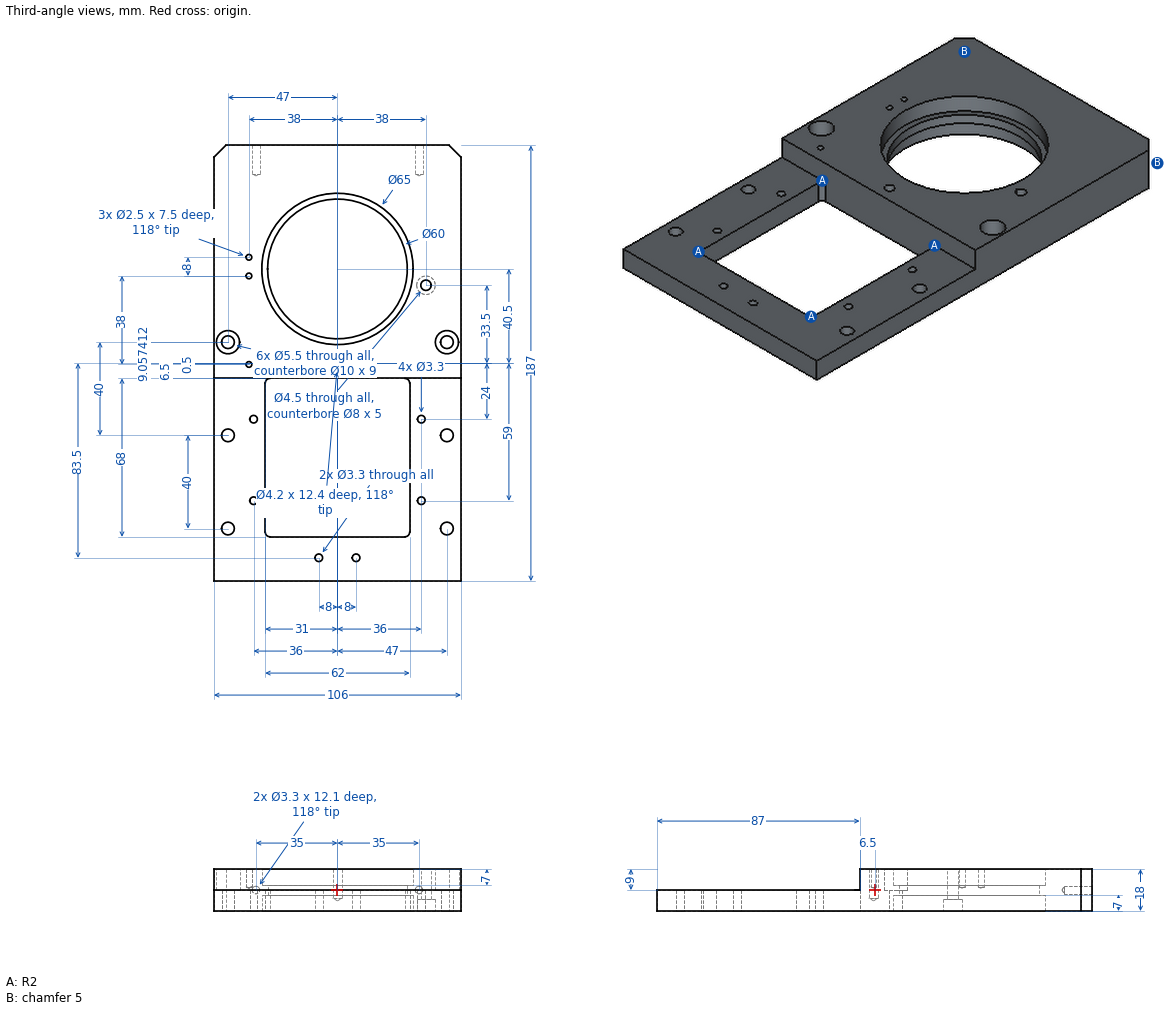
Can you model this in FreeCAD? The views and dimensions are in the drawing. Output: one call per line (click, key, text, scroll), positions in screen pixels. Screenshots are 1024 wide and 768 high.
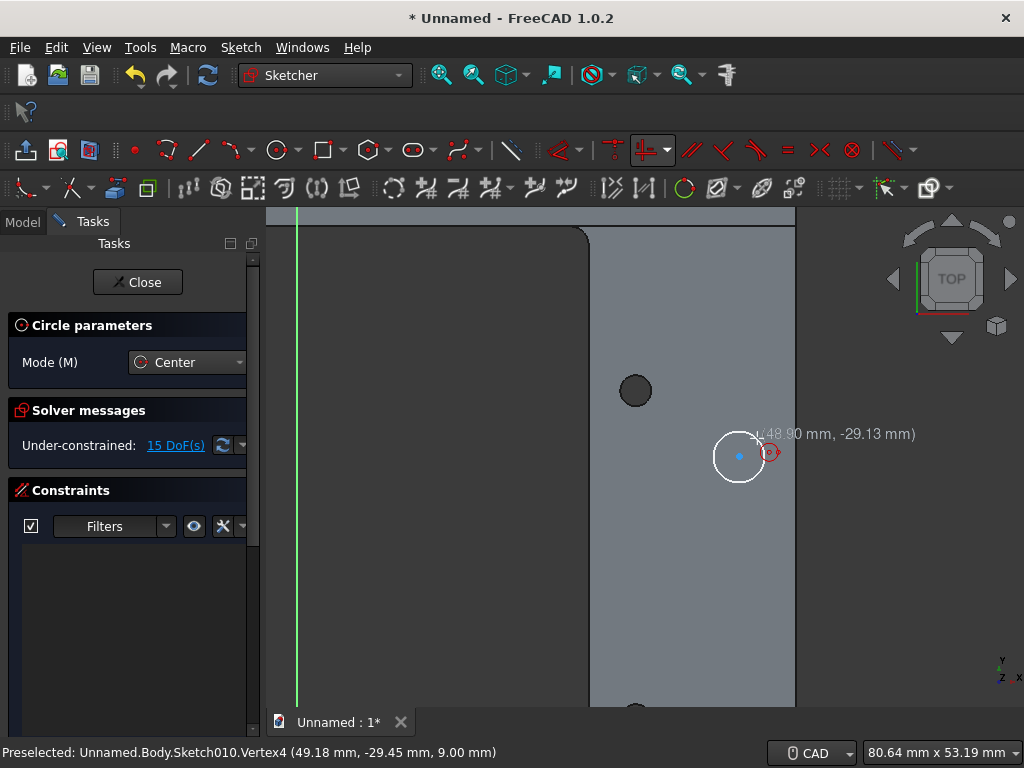
scroll(739, 458, down, 5)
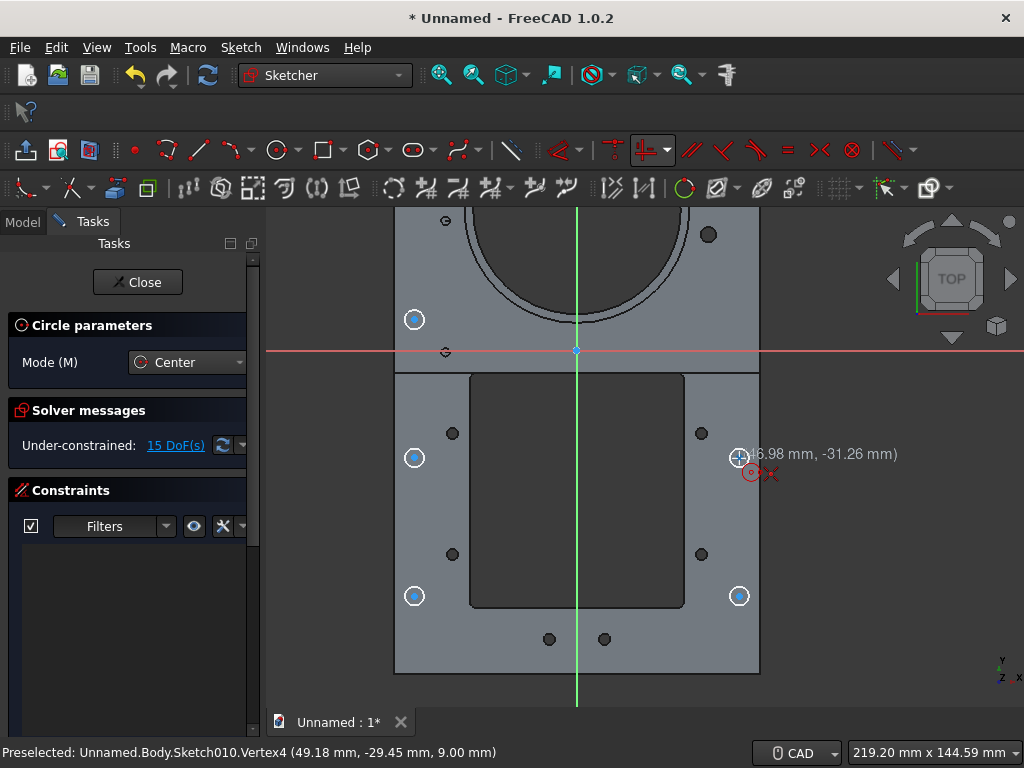
scroll(739, 319, up, 5)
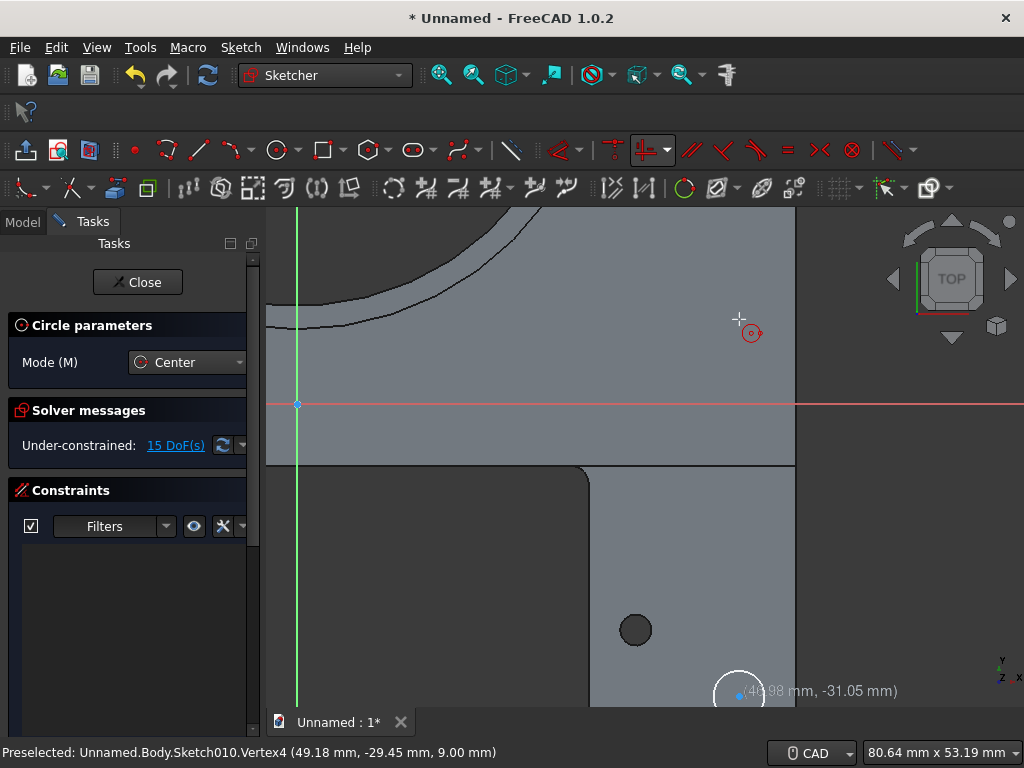
click(739, 319)
click(757, 301)
key(Escape)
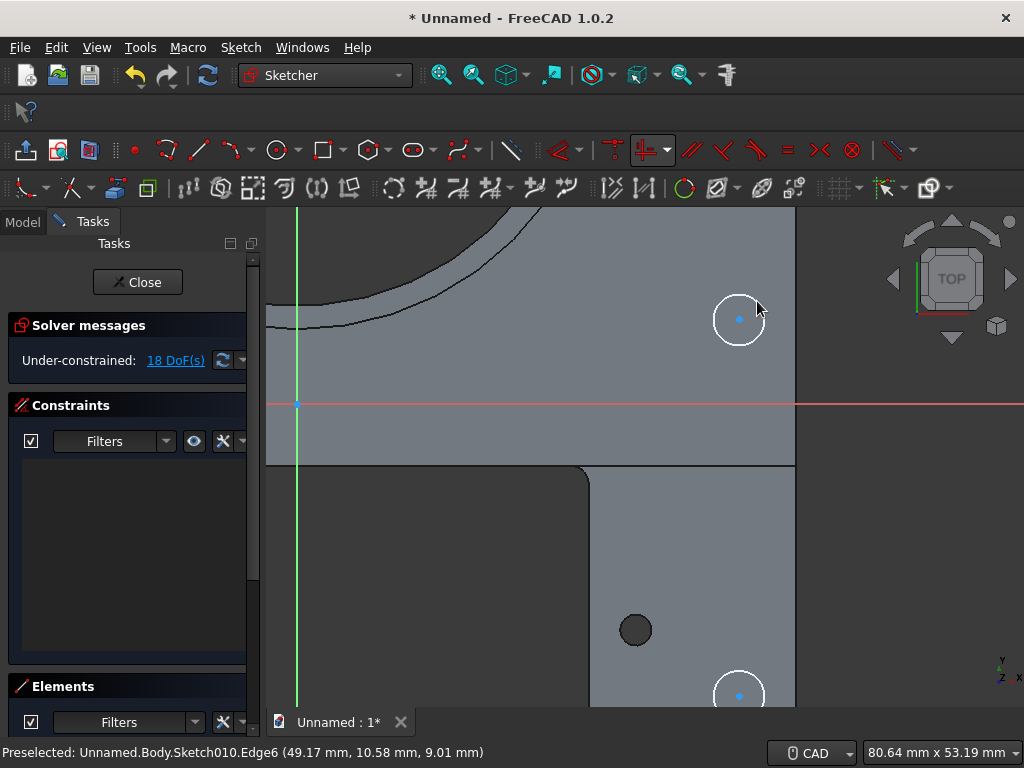
scroll(739, 318, down, 5)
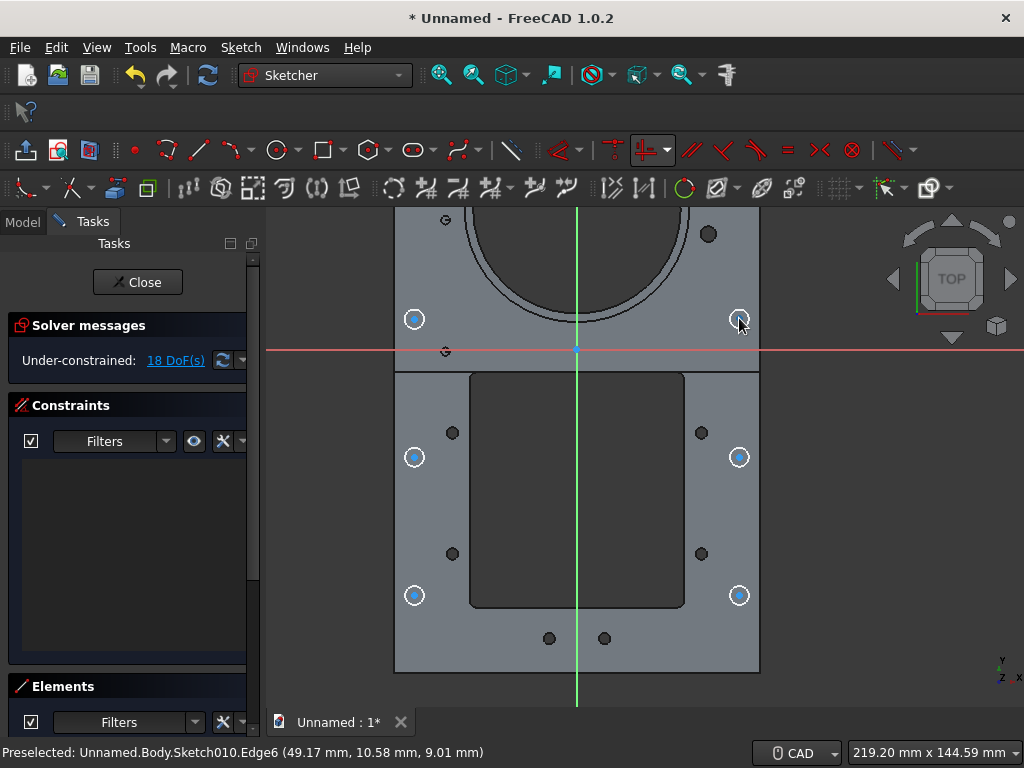
scroll(421, 312, up, 2)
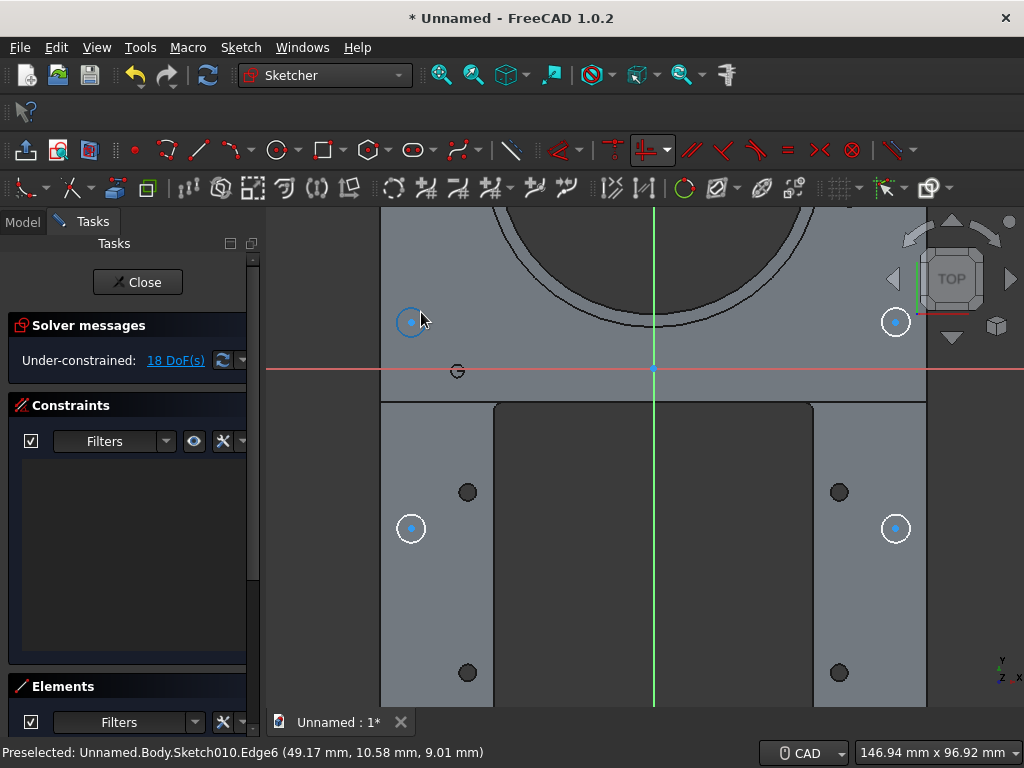
click(421, 312)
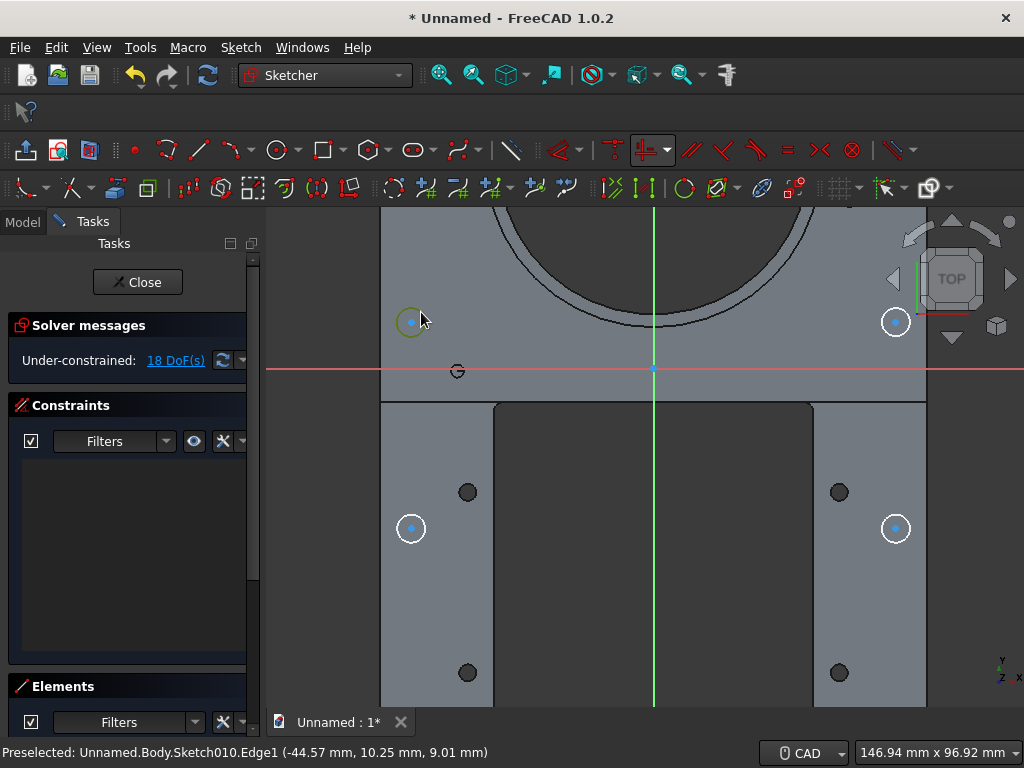
click(421, 519)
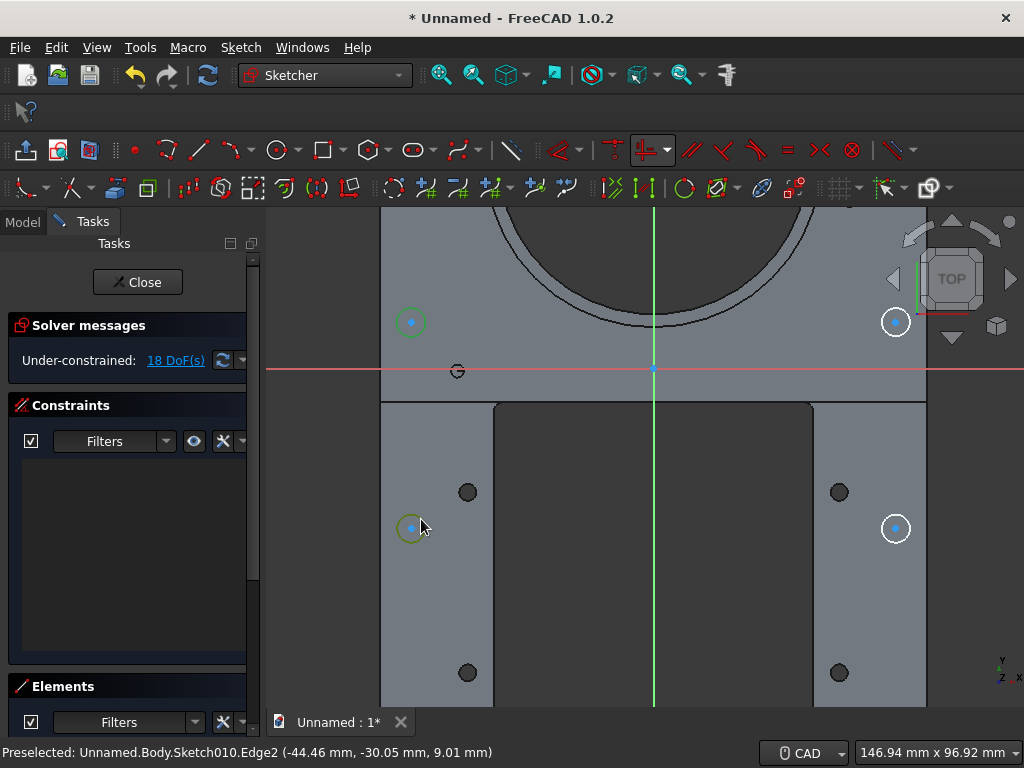
scroll(420, 312, down, 2)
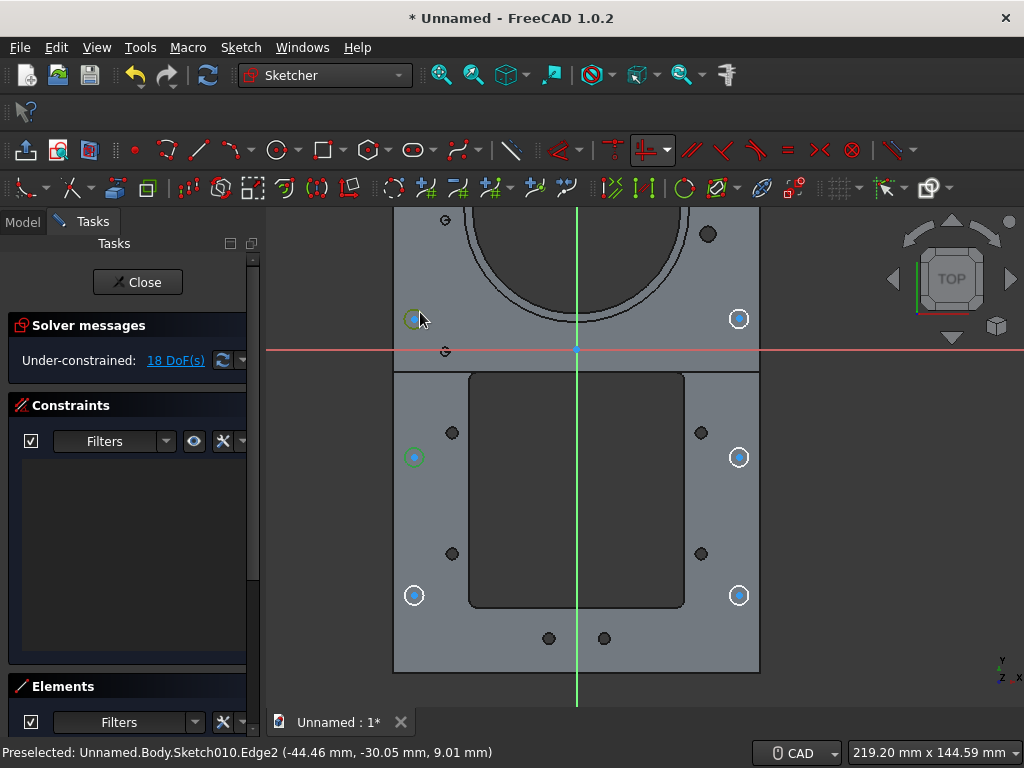
scroll(421, 589, up, 2)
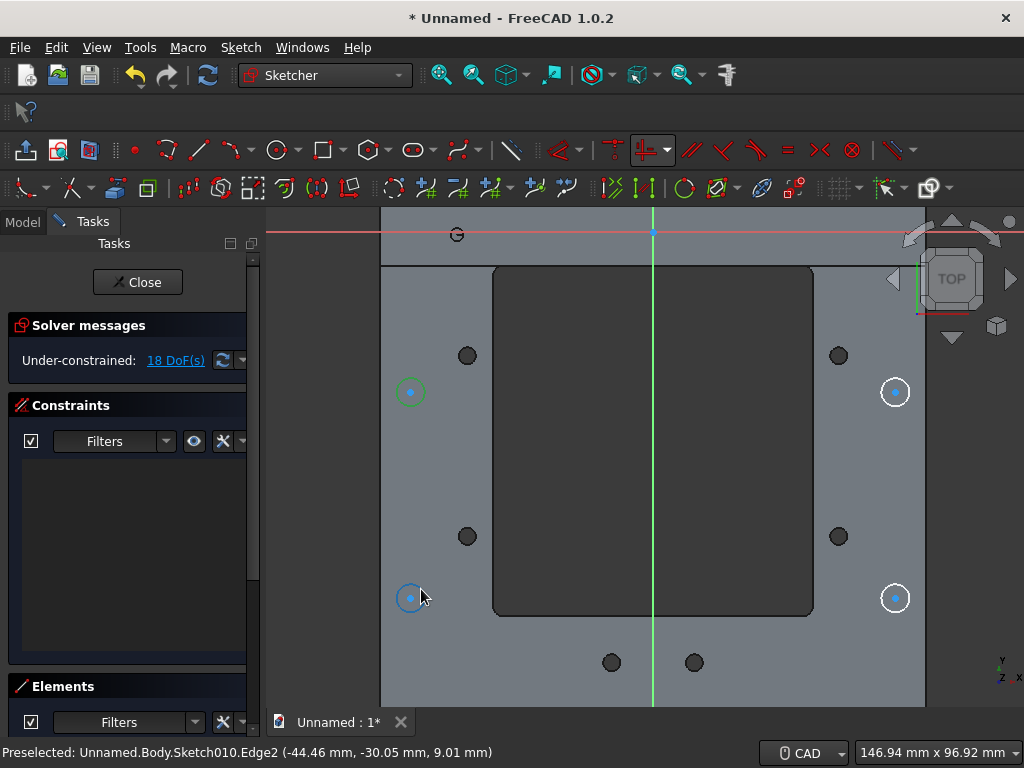
click(421, 588)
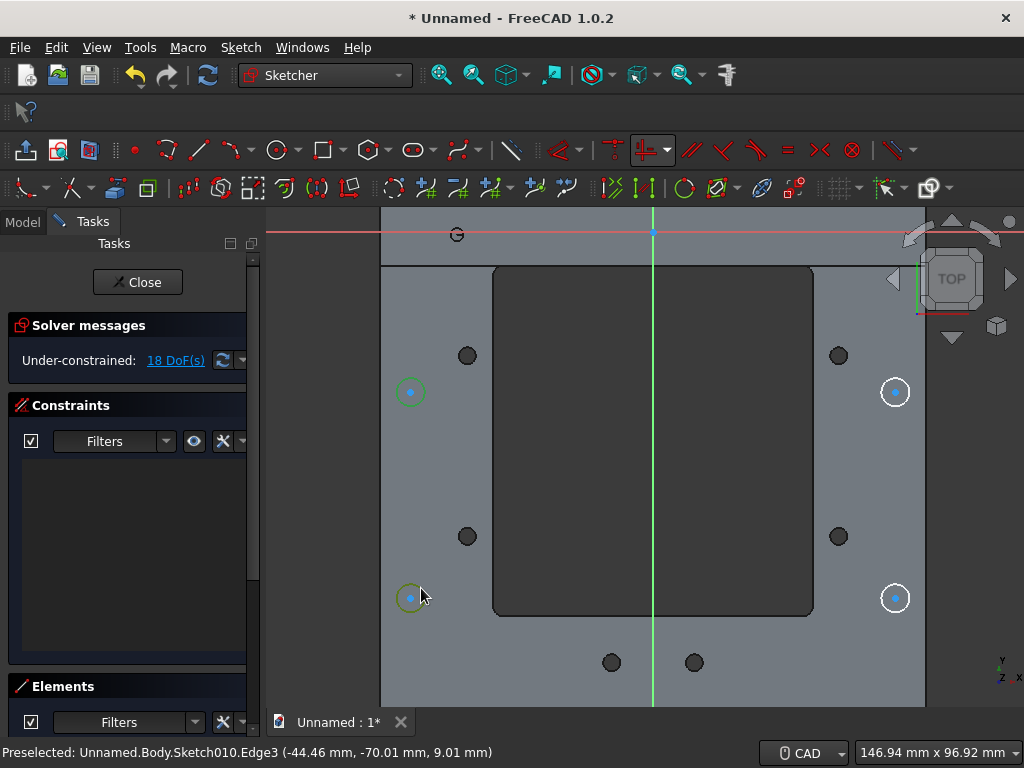
scroll(421, 590, down, 2)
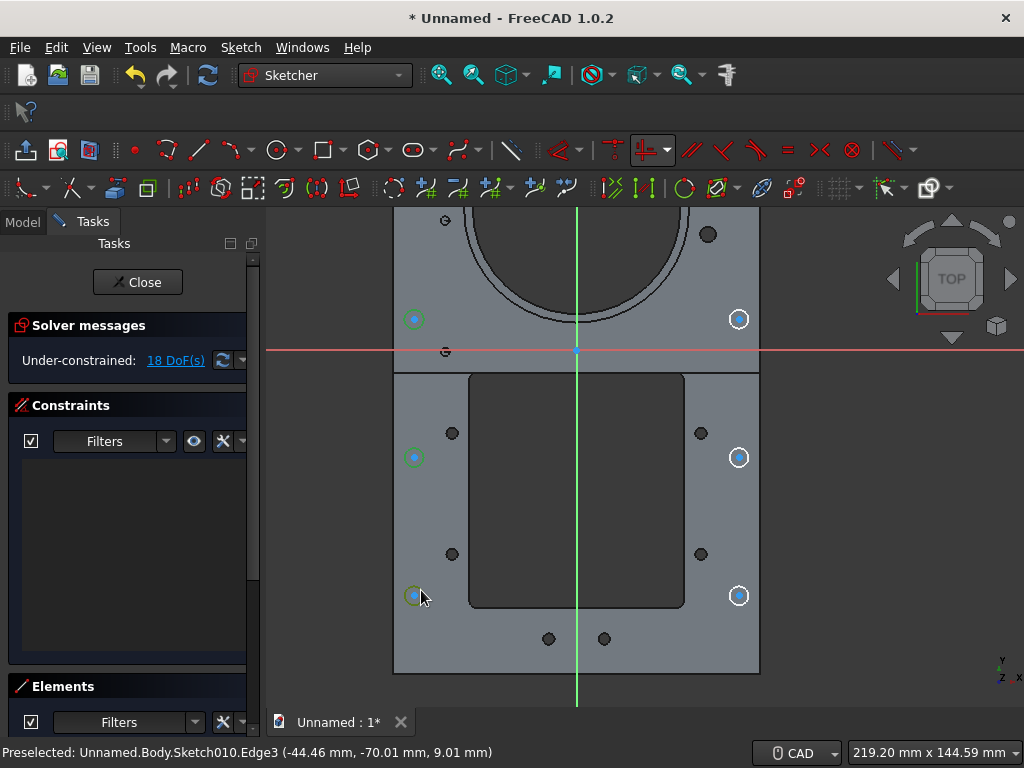
scroll(746, 589, up, 2)